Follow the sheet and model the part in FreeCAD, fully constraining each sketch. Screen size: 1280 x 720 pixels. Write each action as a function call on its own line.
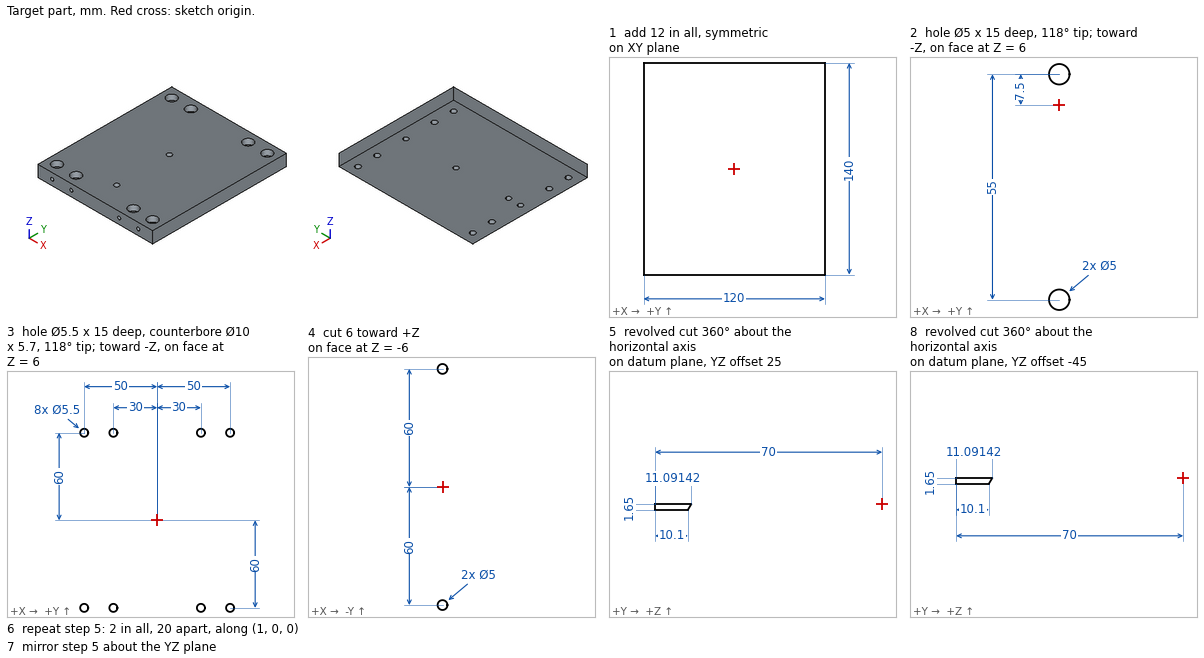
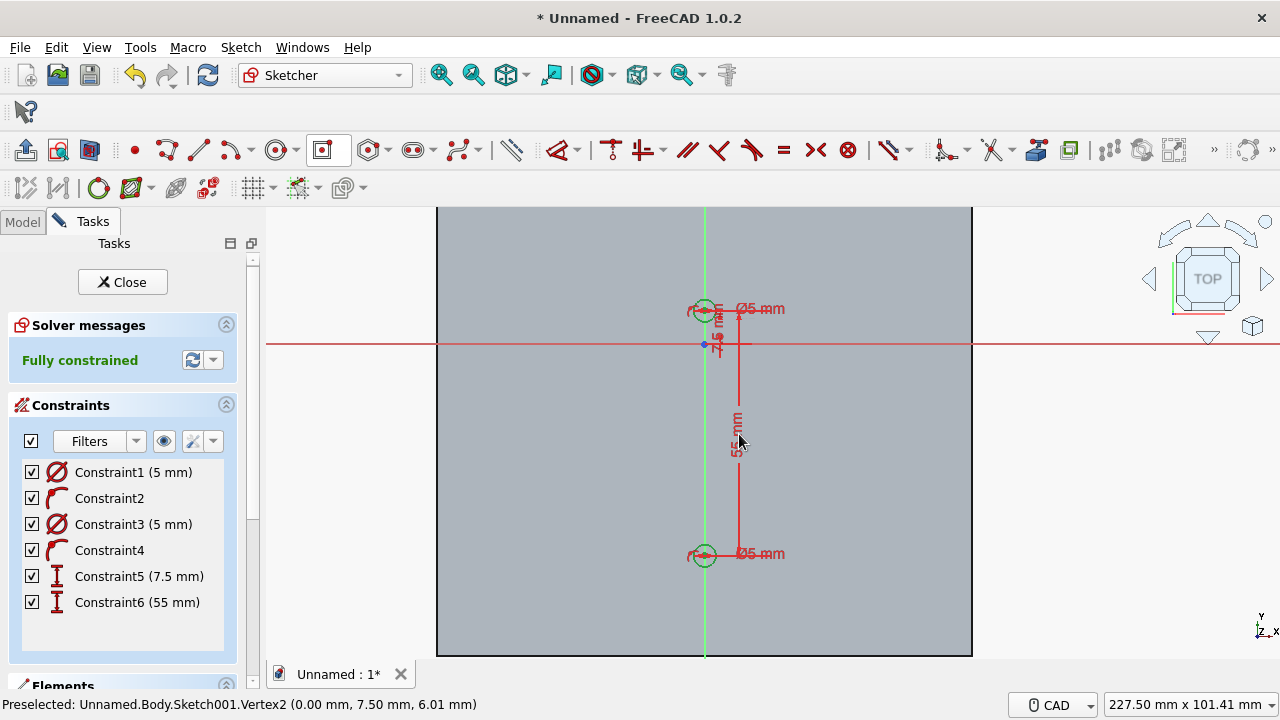
click(123, 282)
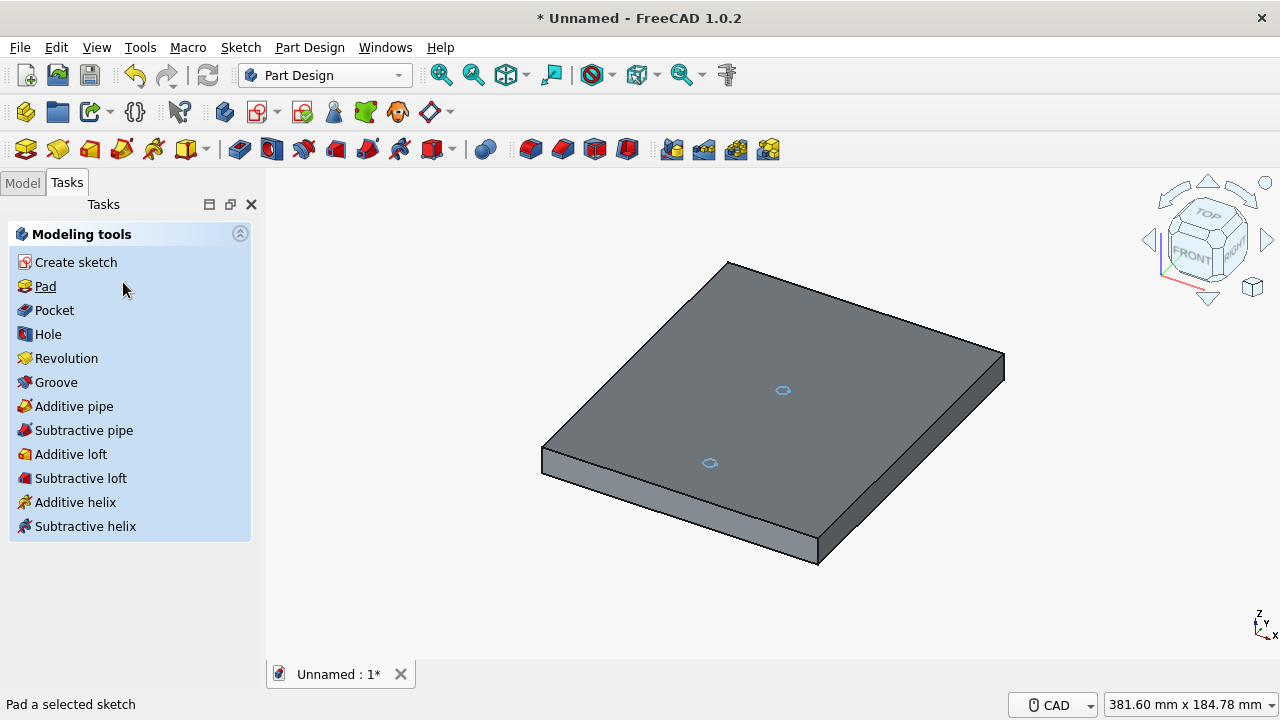
click(272, 150)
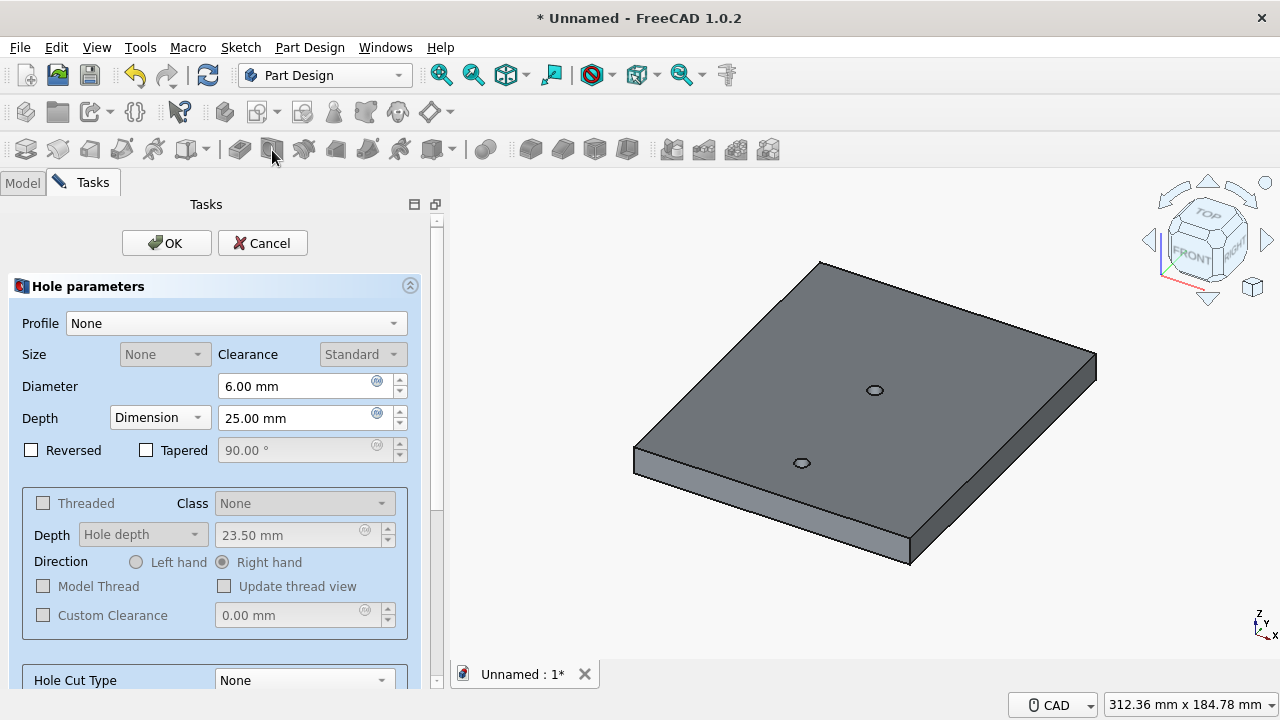
triple_click(305, 386)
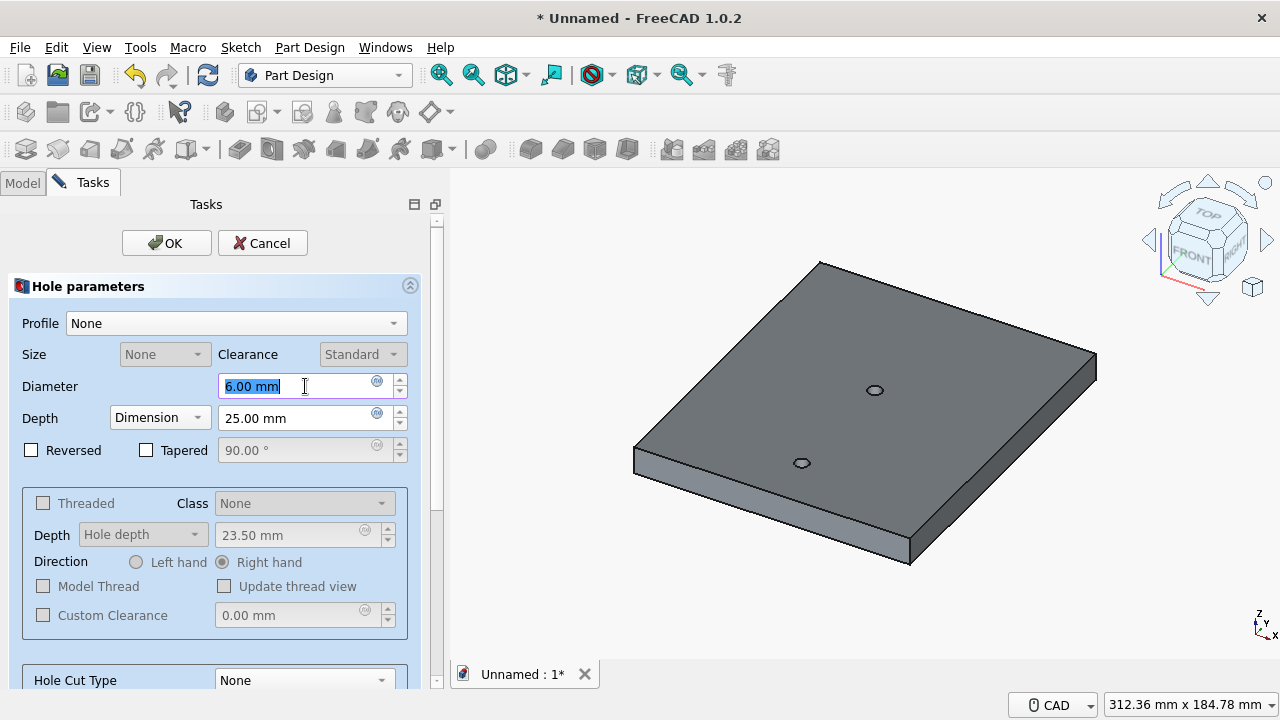
text(5)
key(Tab)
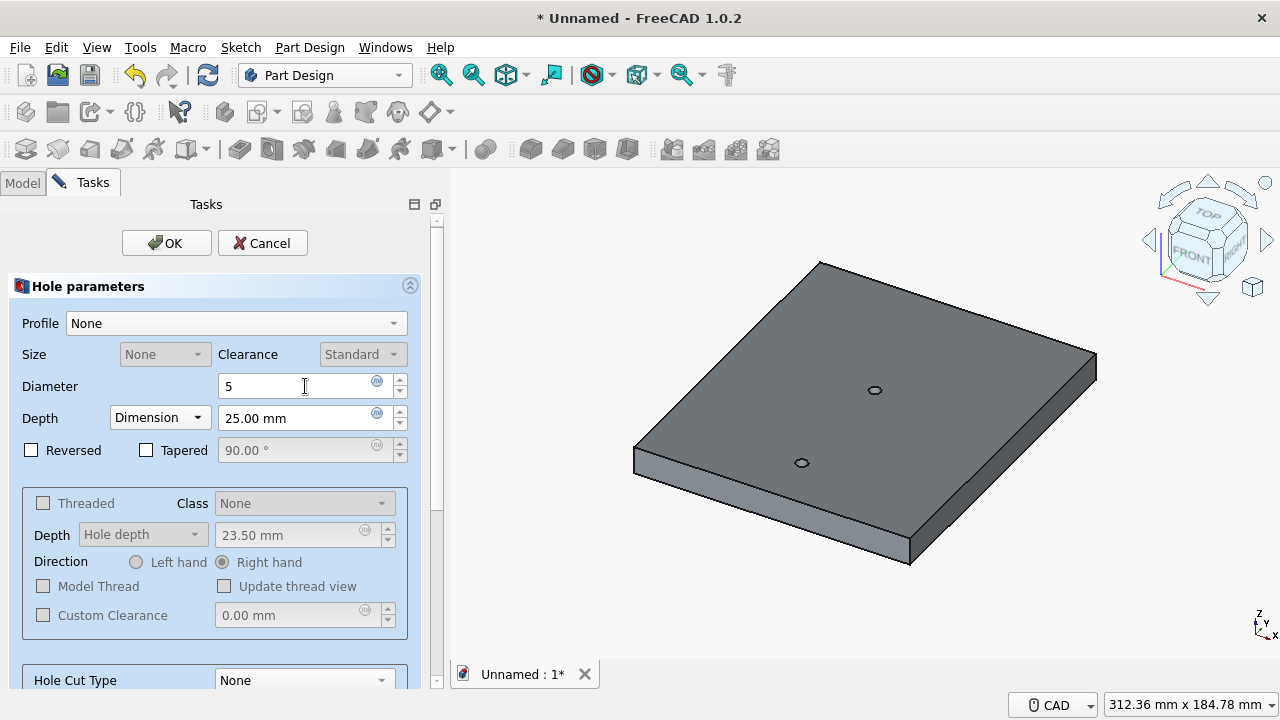
triple_click(305, 418)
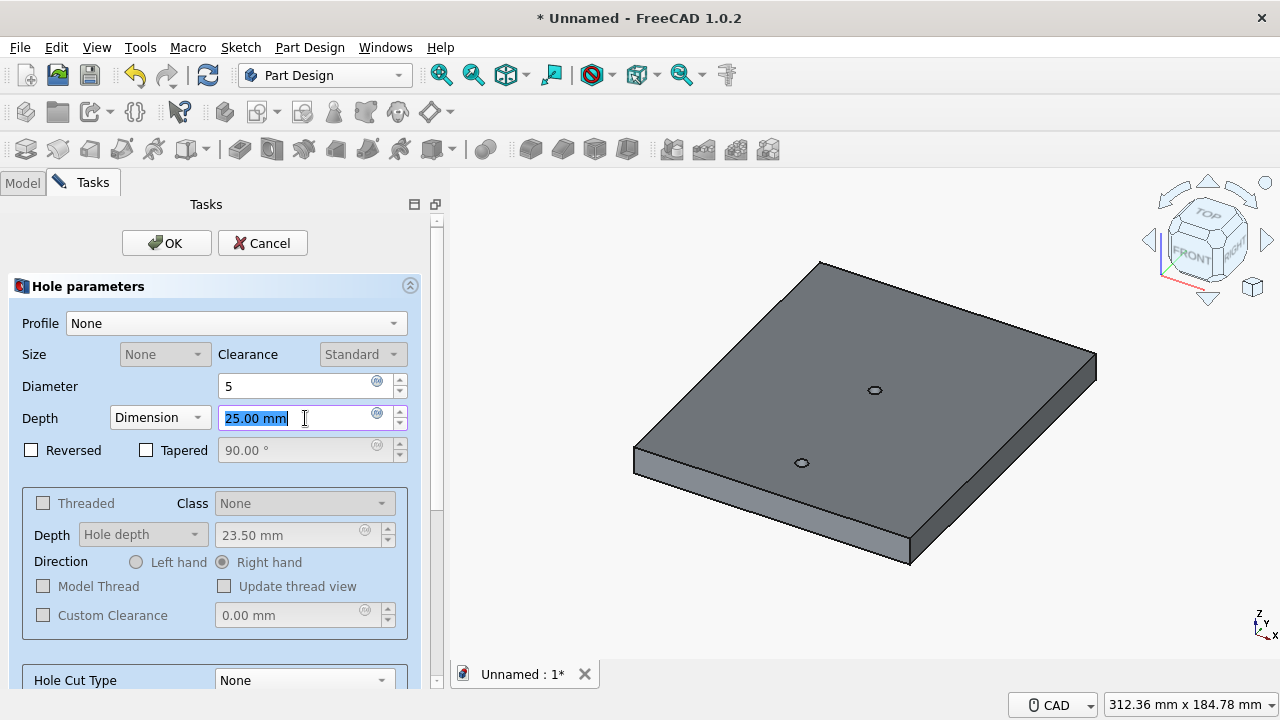
text(15)
key(Tab)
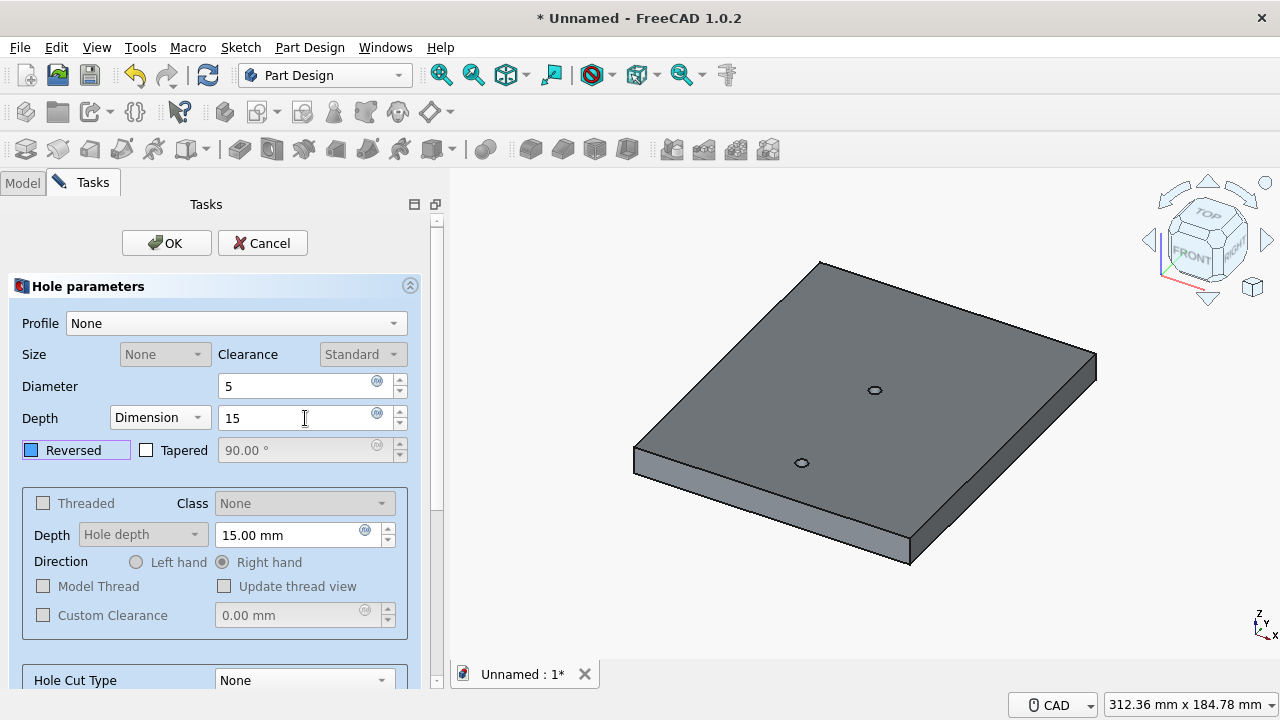
click(167, 243)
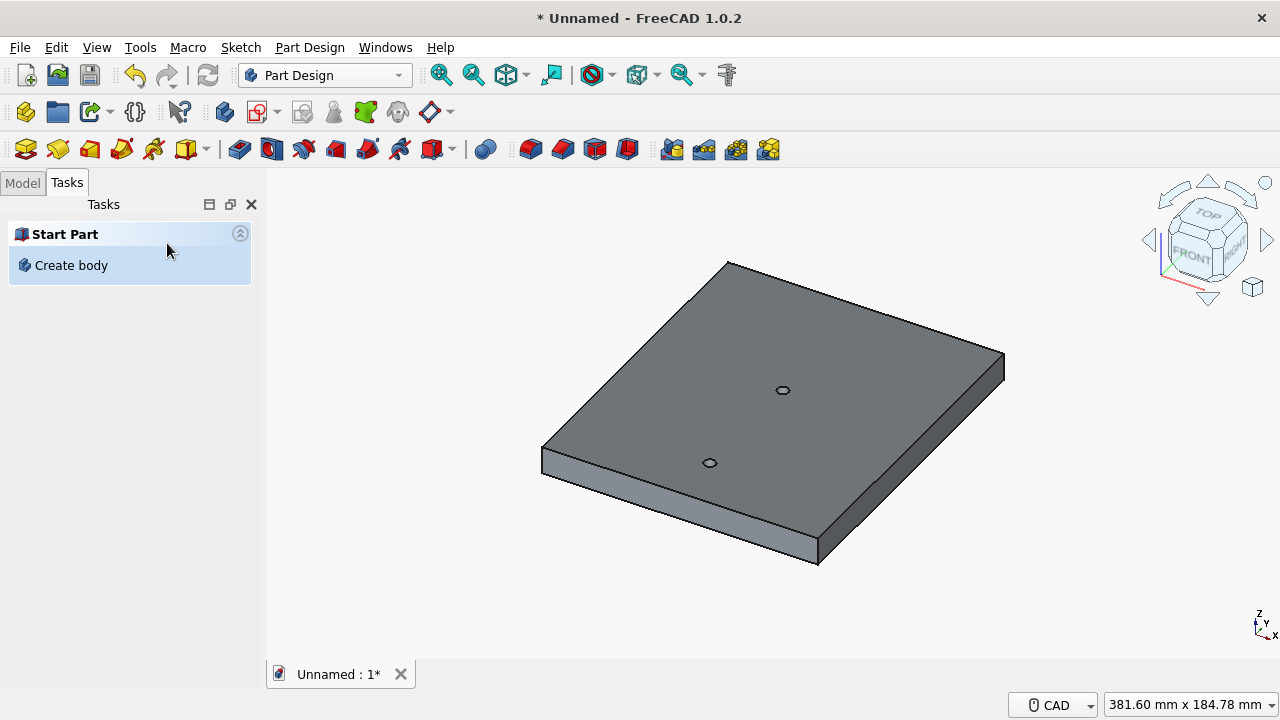
click(866, 360)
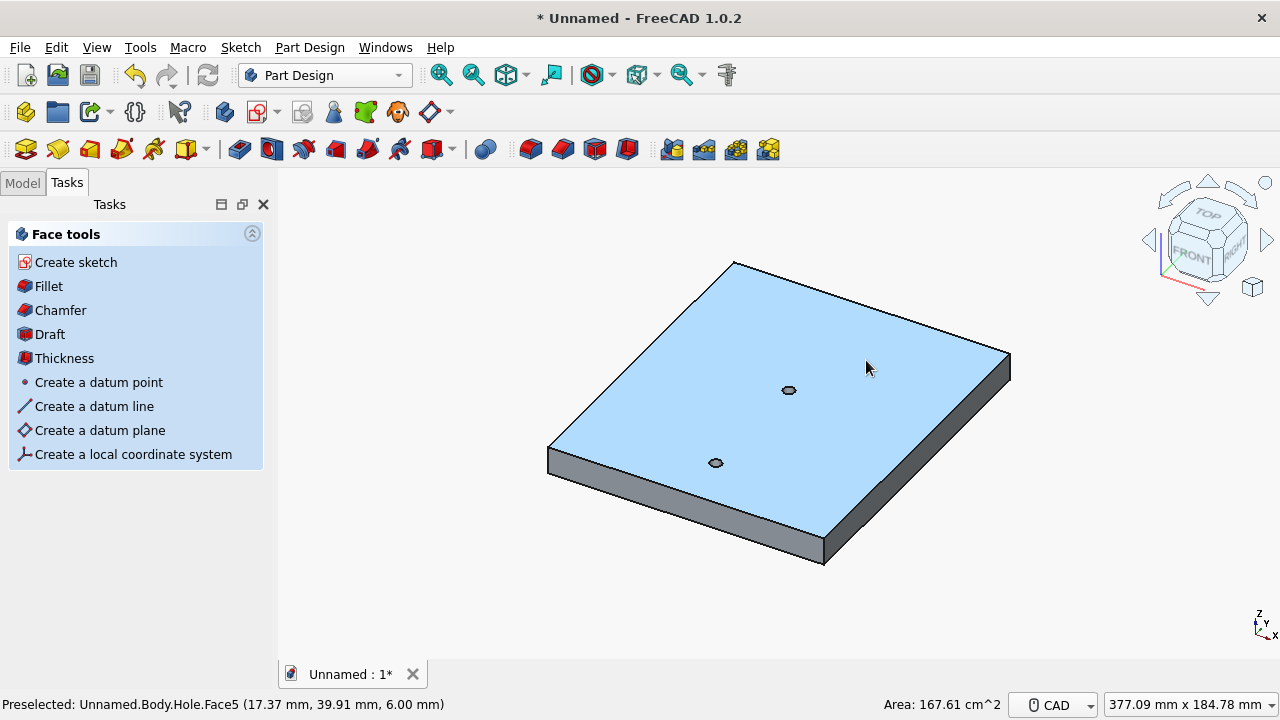
click(258, 112)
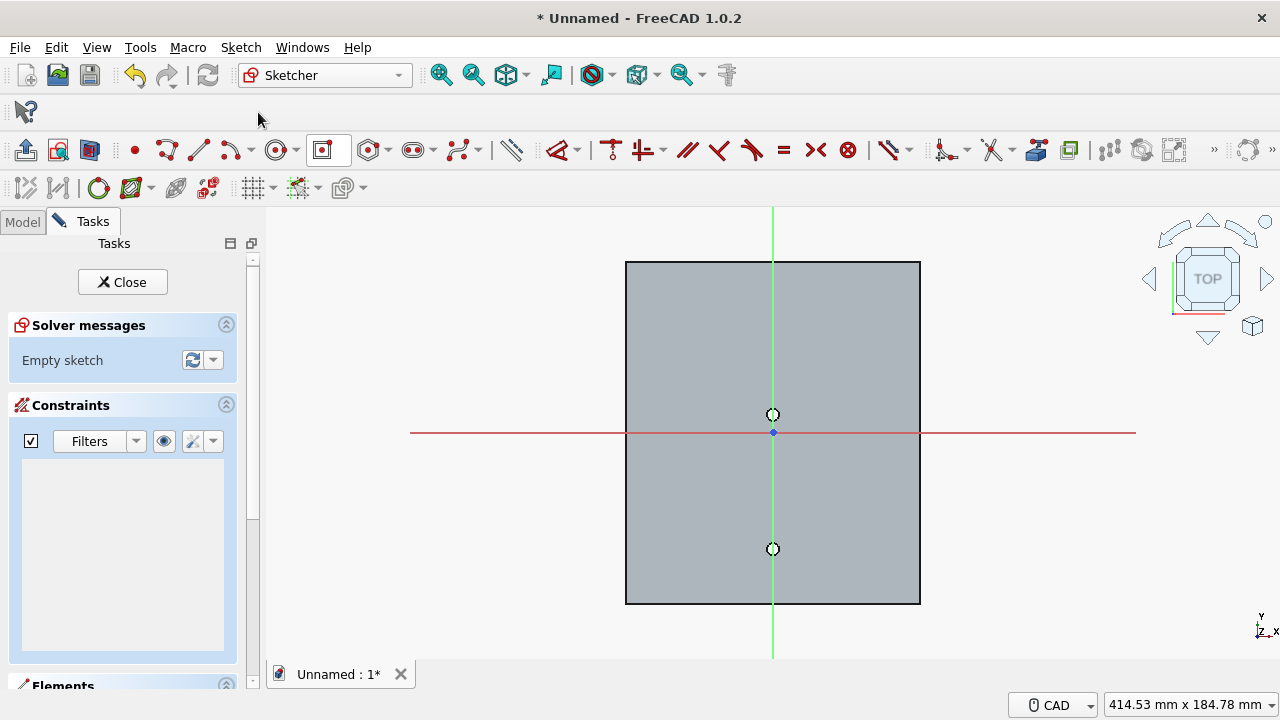
key(g)
key(c)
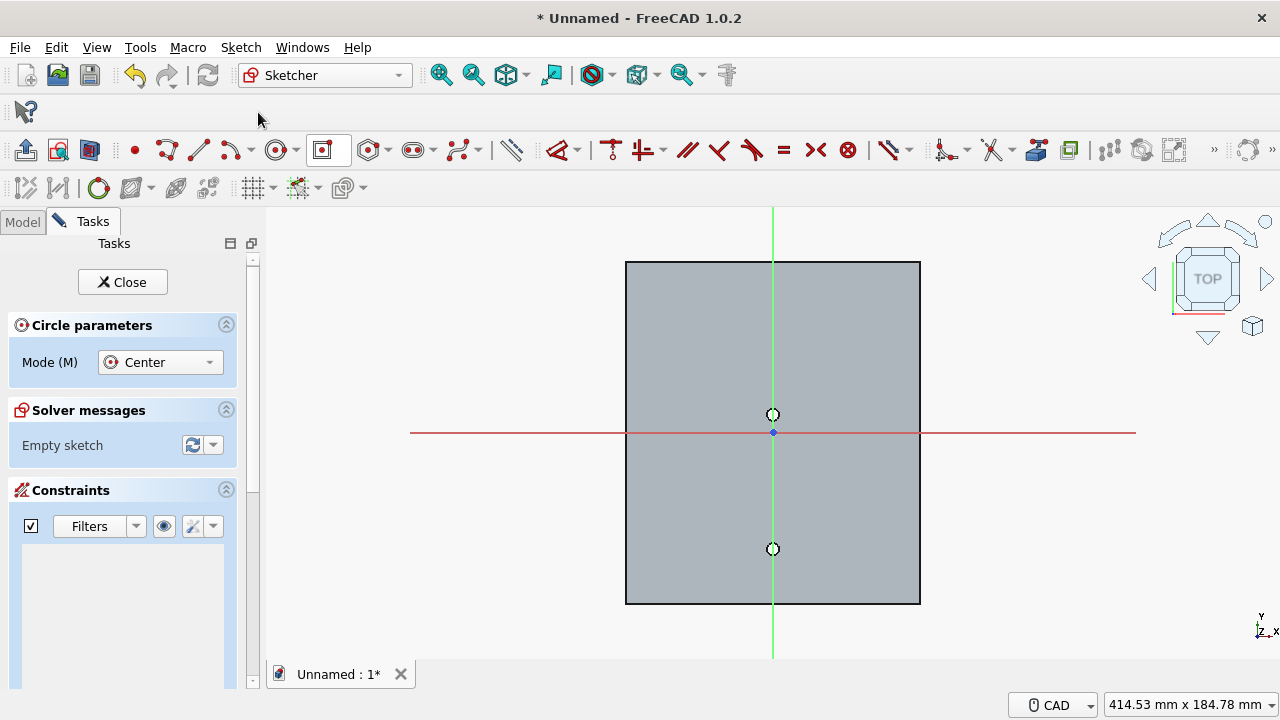
scroll(651, 286, up, 7)